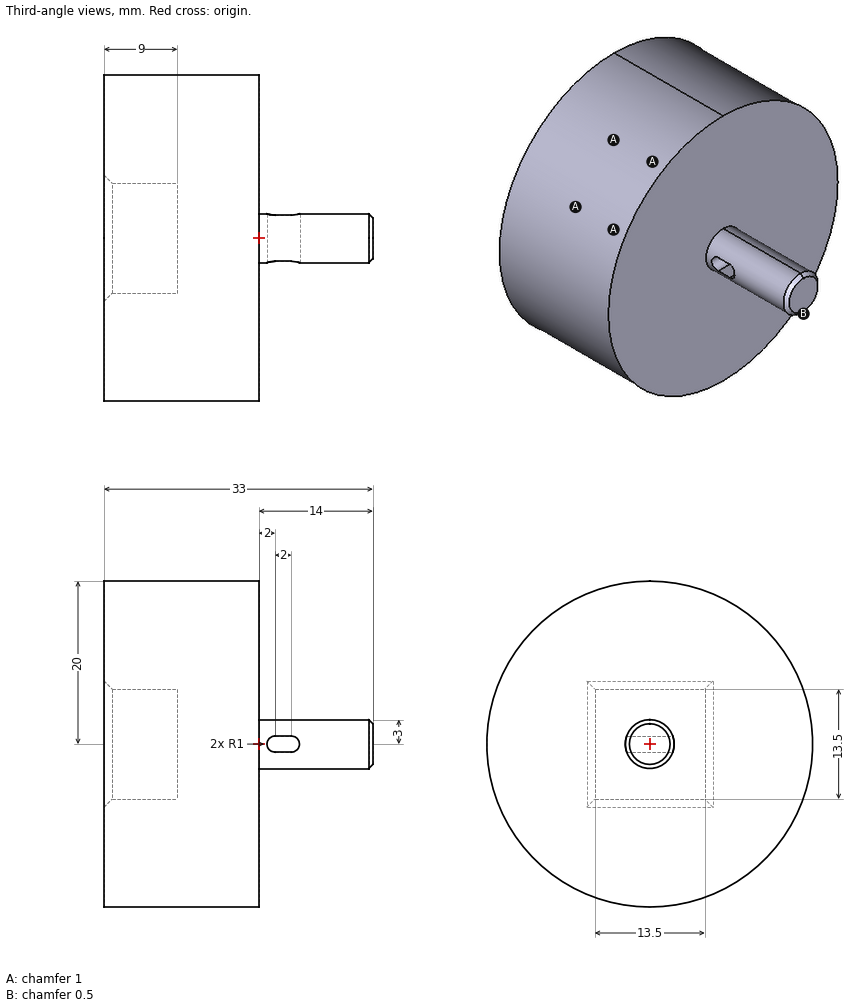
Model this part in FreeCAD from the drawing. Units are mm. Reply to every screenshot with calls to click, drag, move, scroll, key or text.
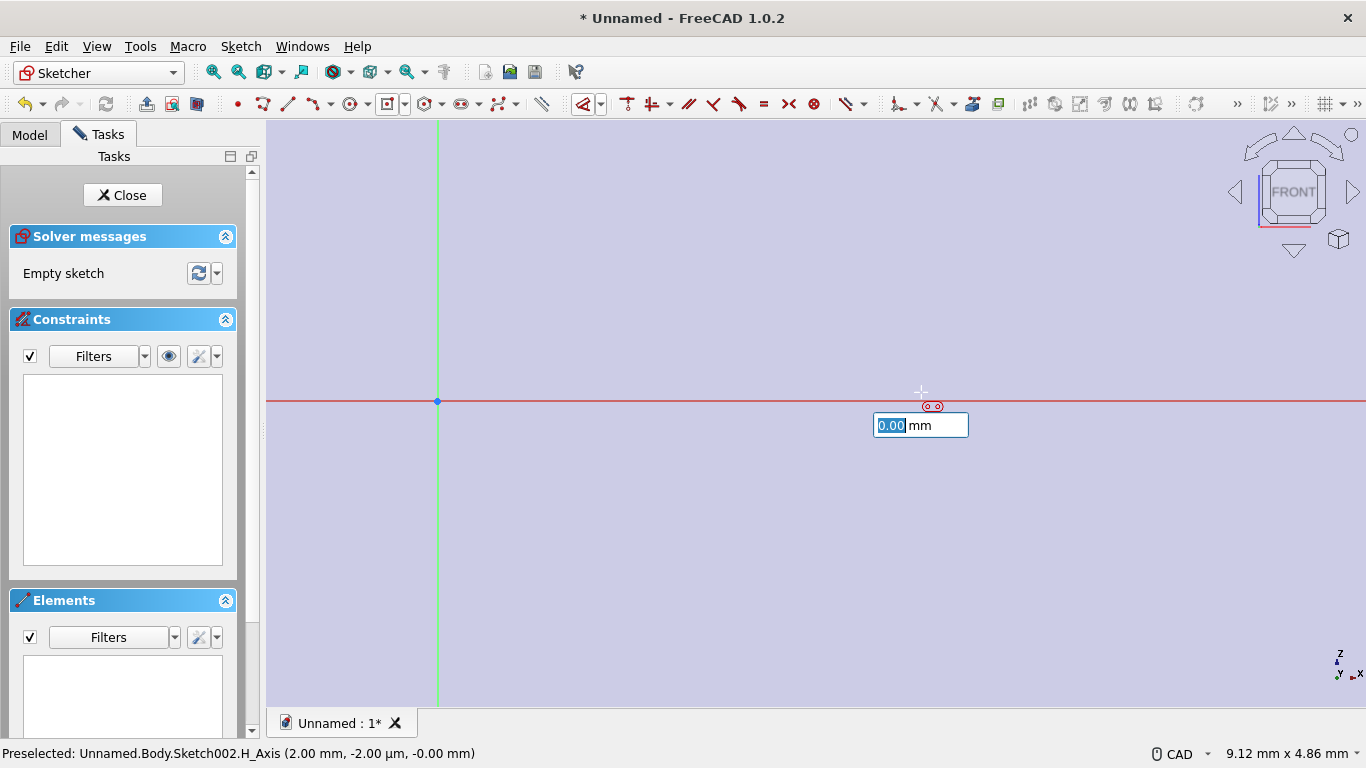
click(800, 522)
key(Escape)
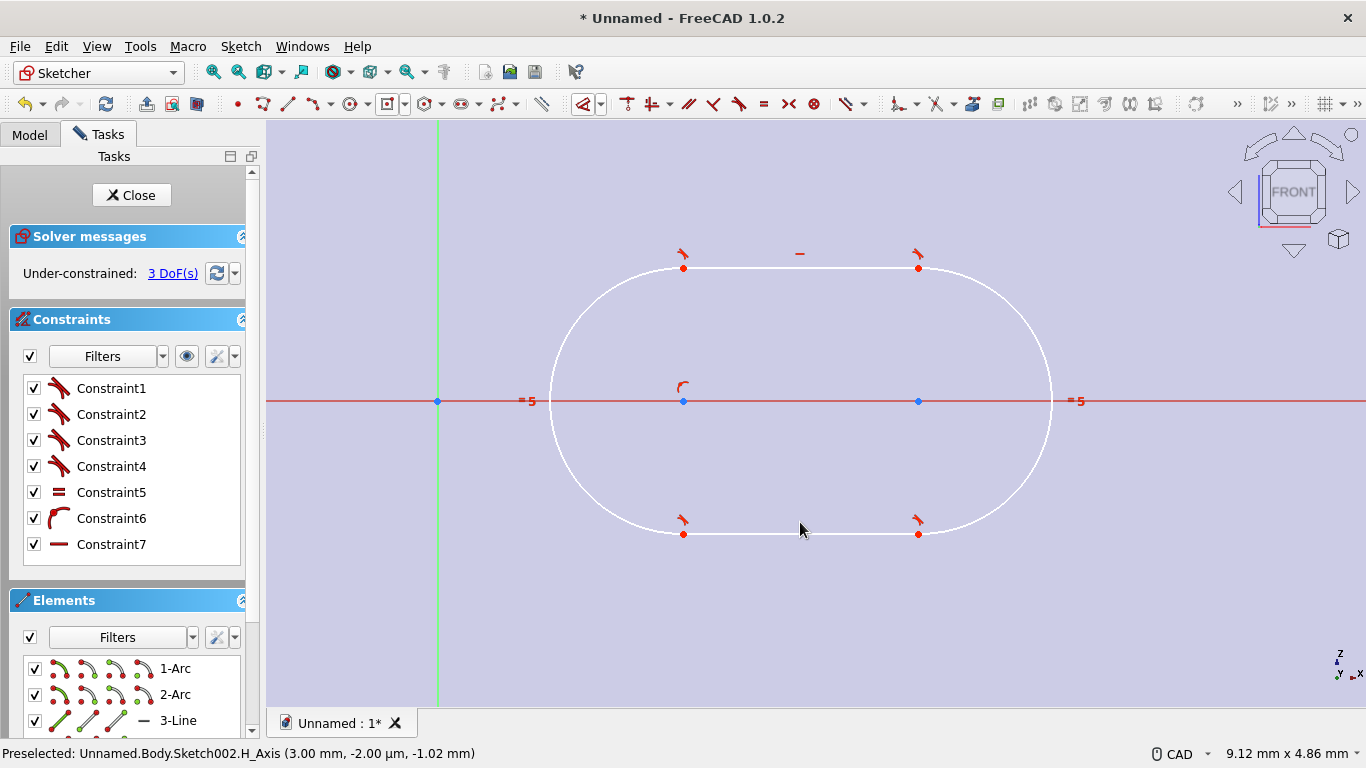
click(575, 323)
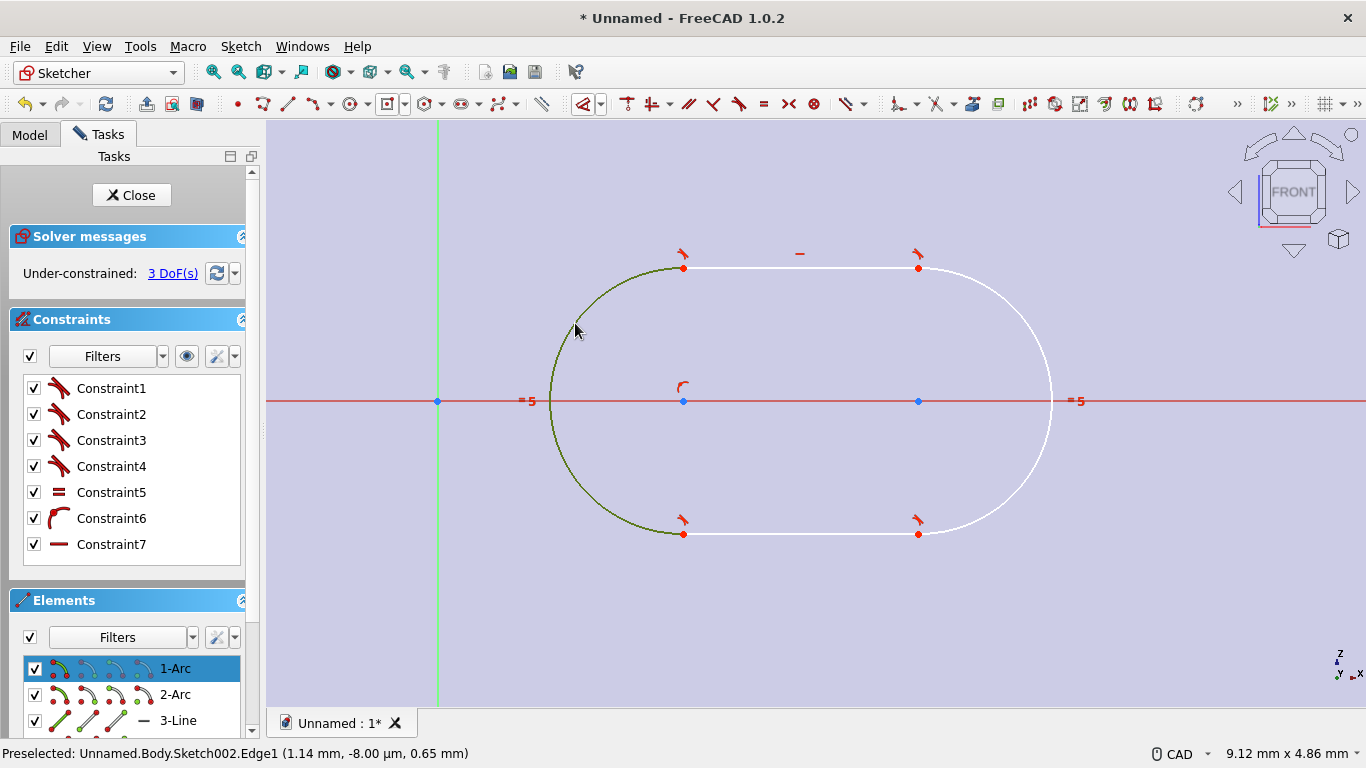
click(600, 104)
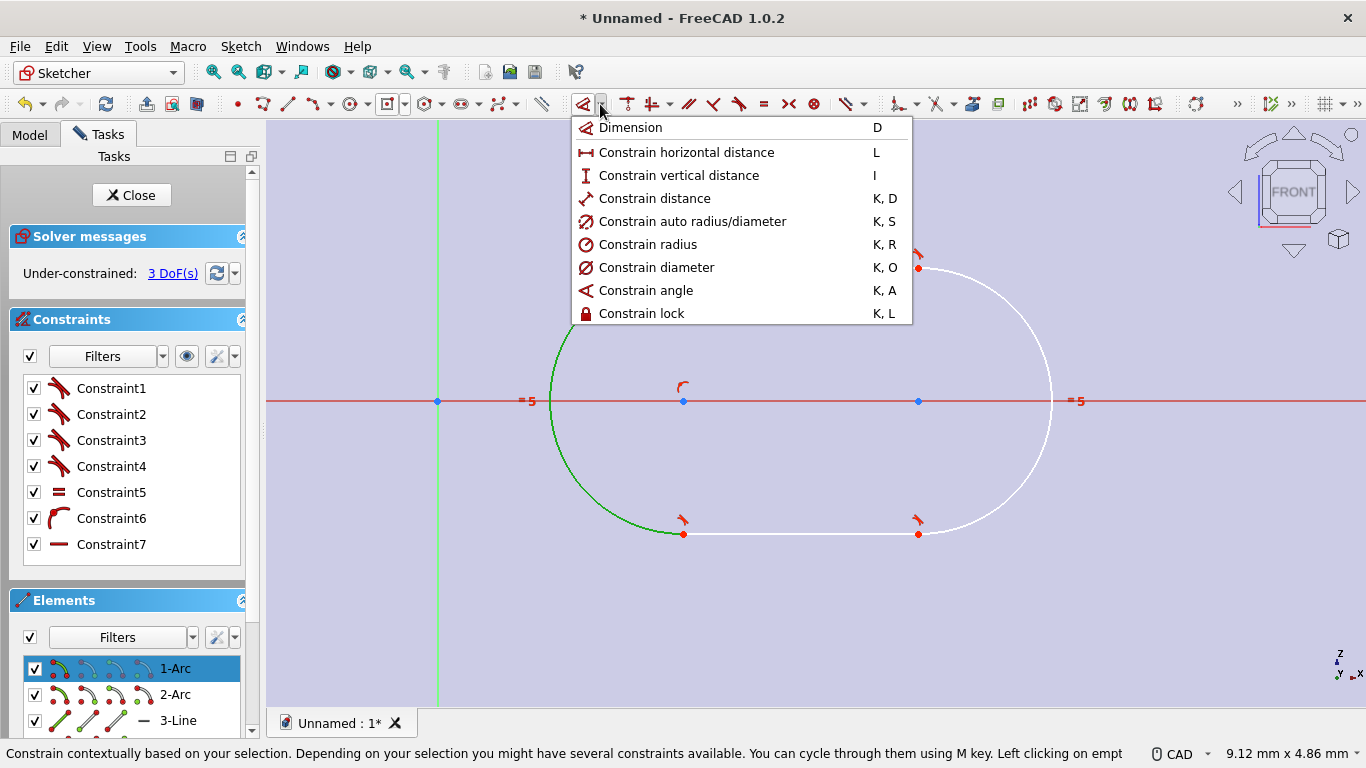
click(742, 244)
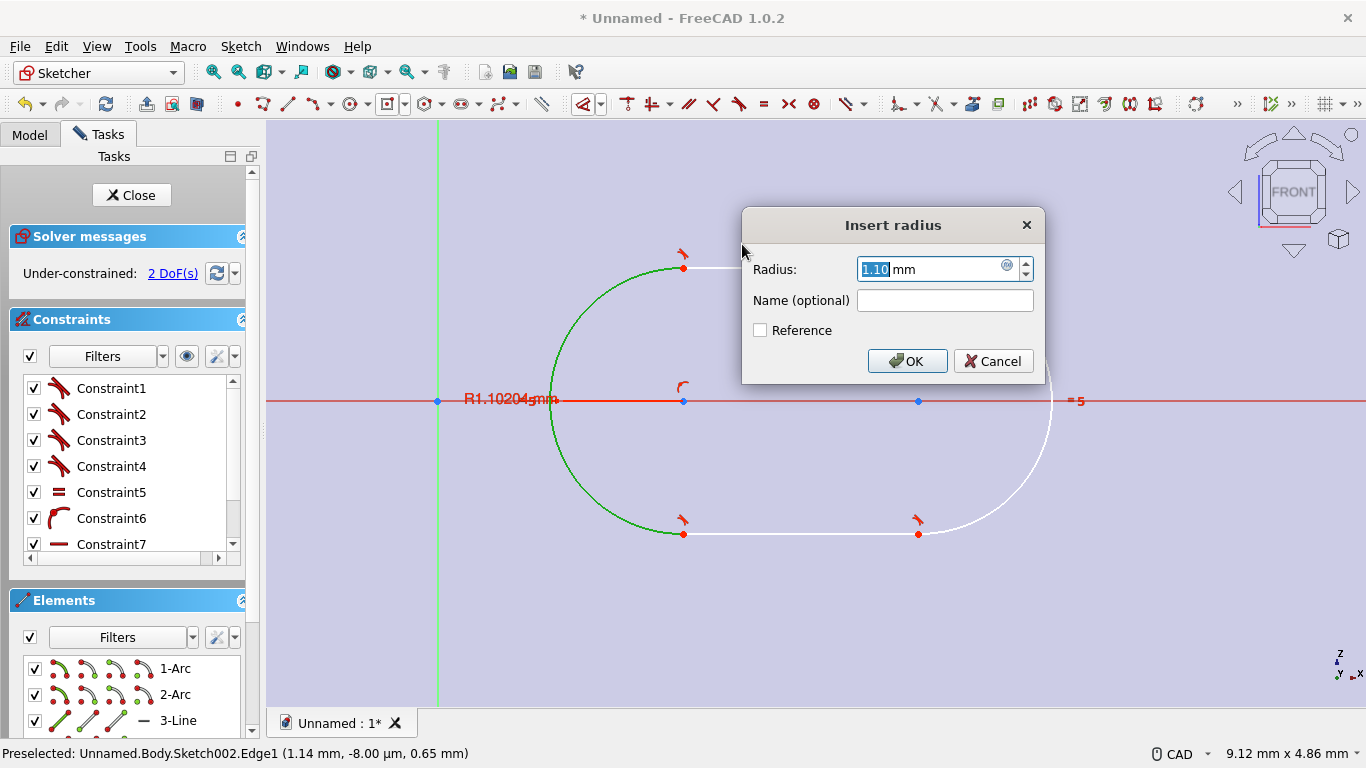
text(1)
key(Return)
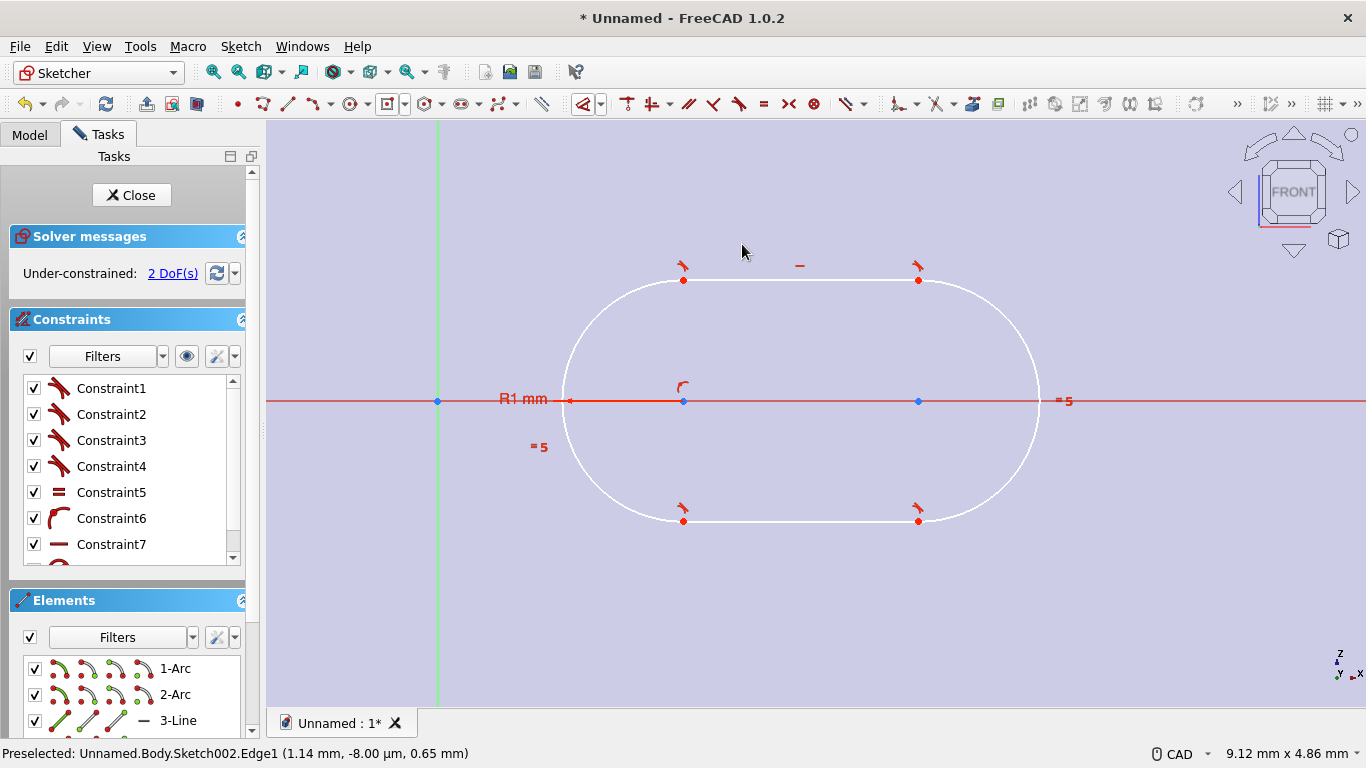
click(754, 280)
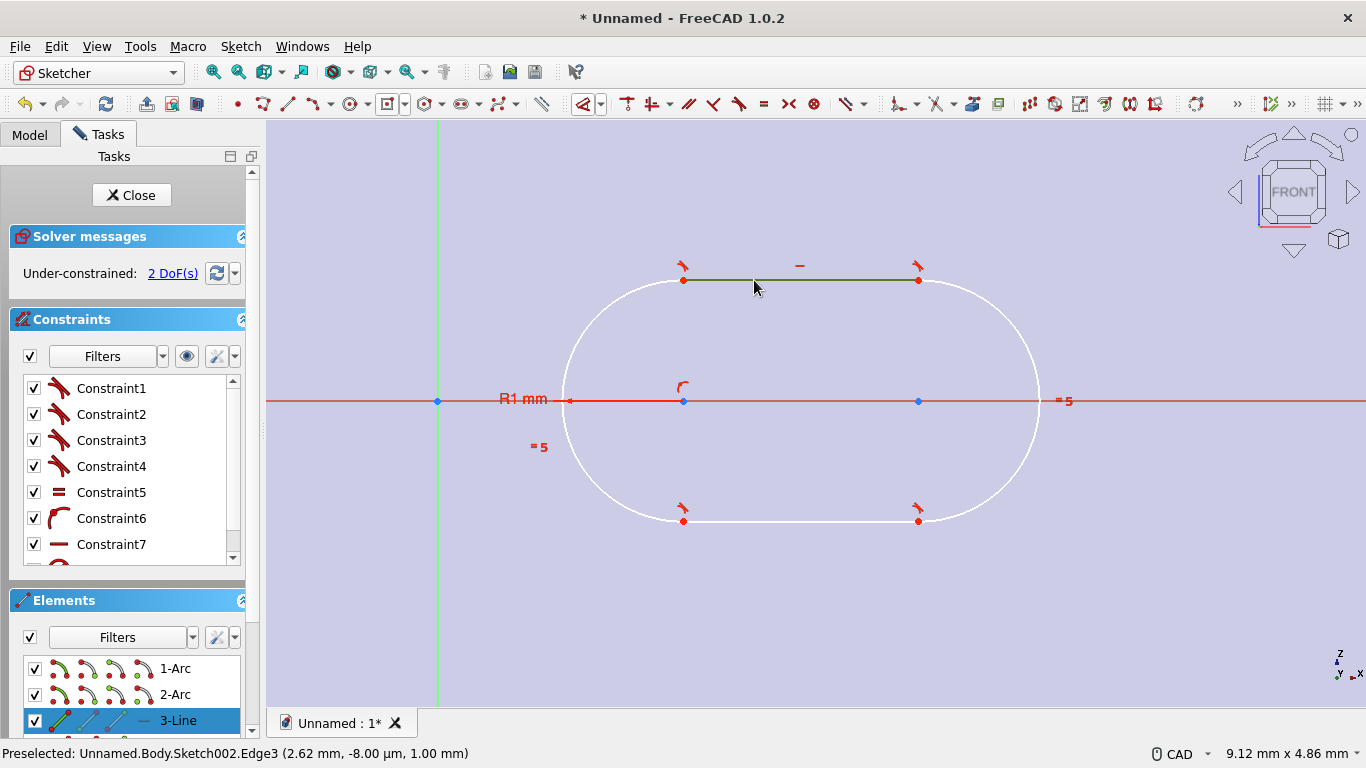
key(l)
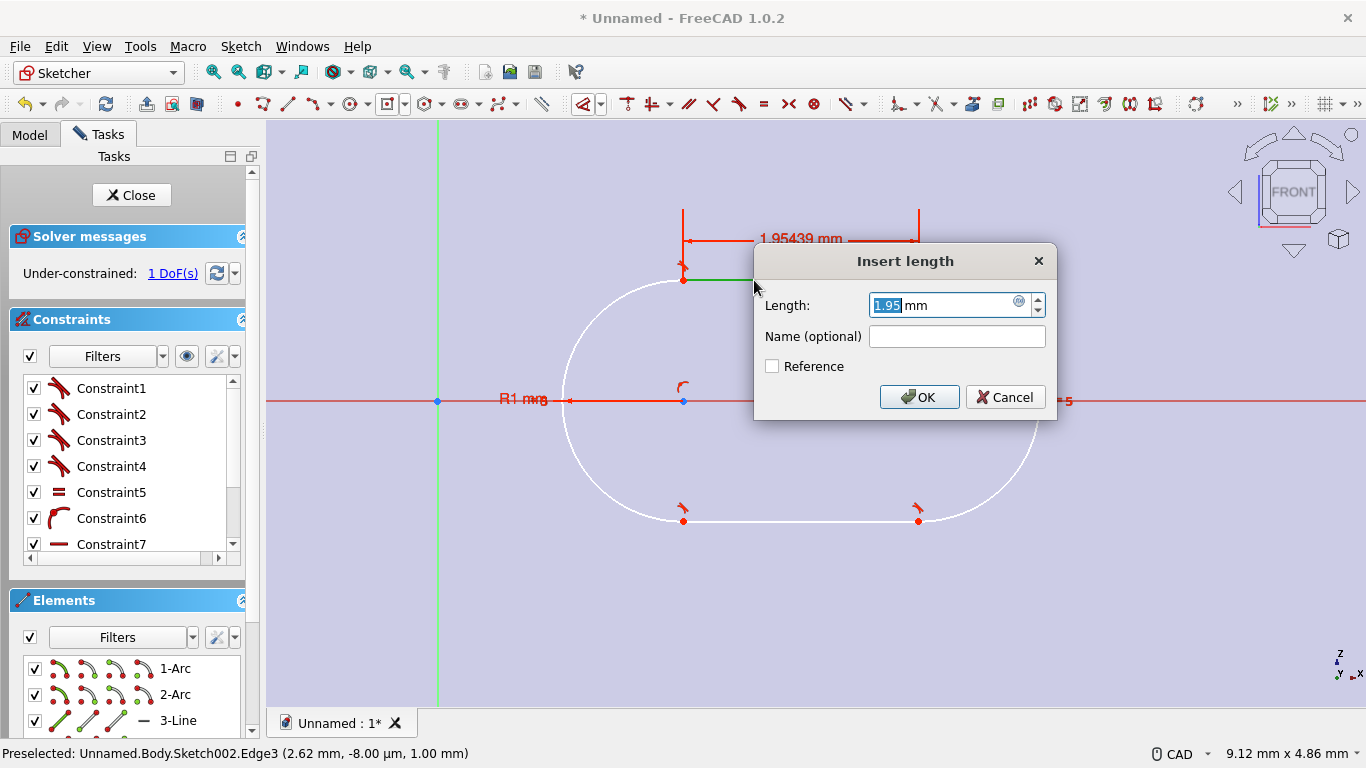
text(2)
key(Return)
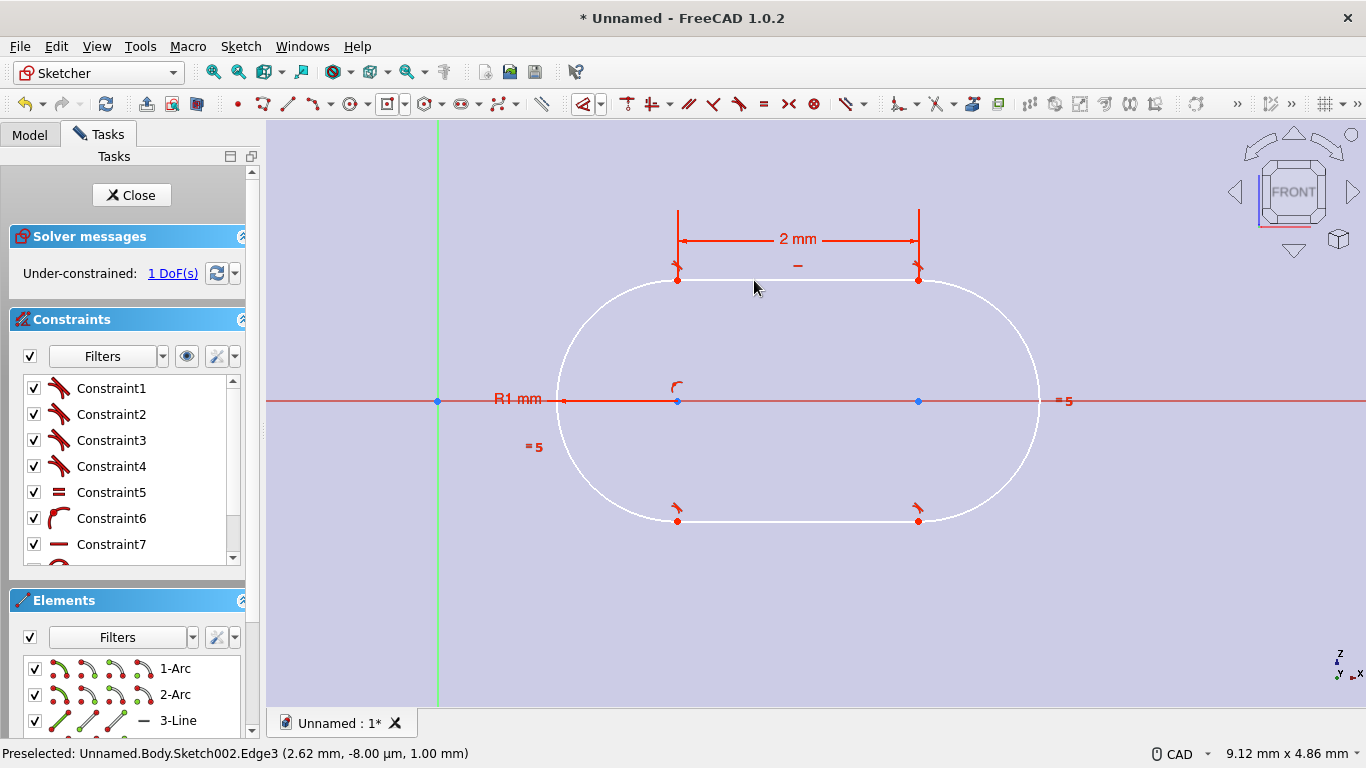
click(678, 280)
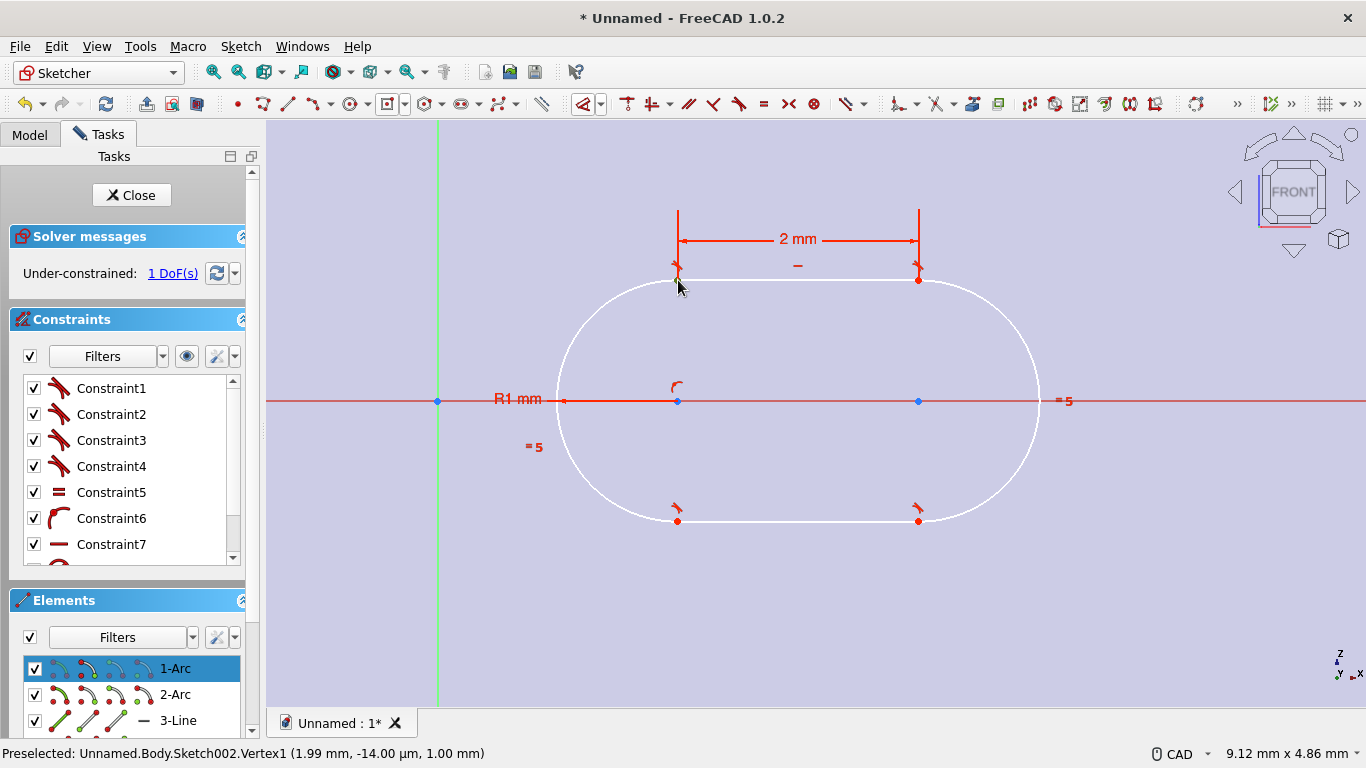
key(l)